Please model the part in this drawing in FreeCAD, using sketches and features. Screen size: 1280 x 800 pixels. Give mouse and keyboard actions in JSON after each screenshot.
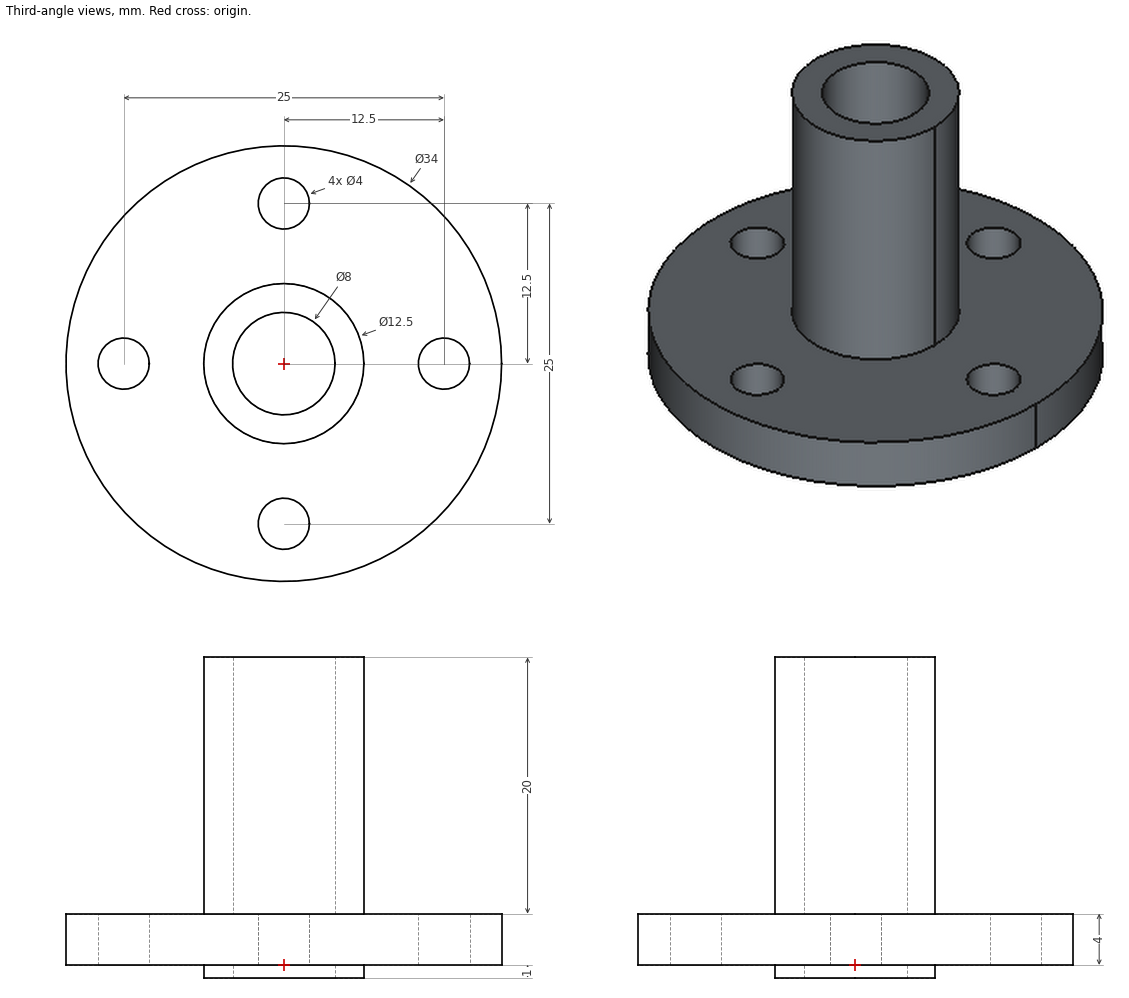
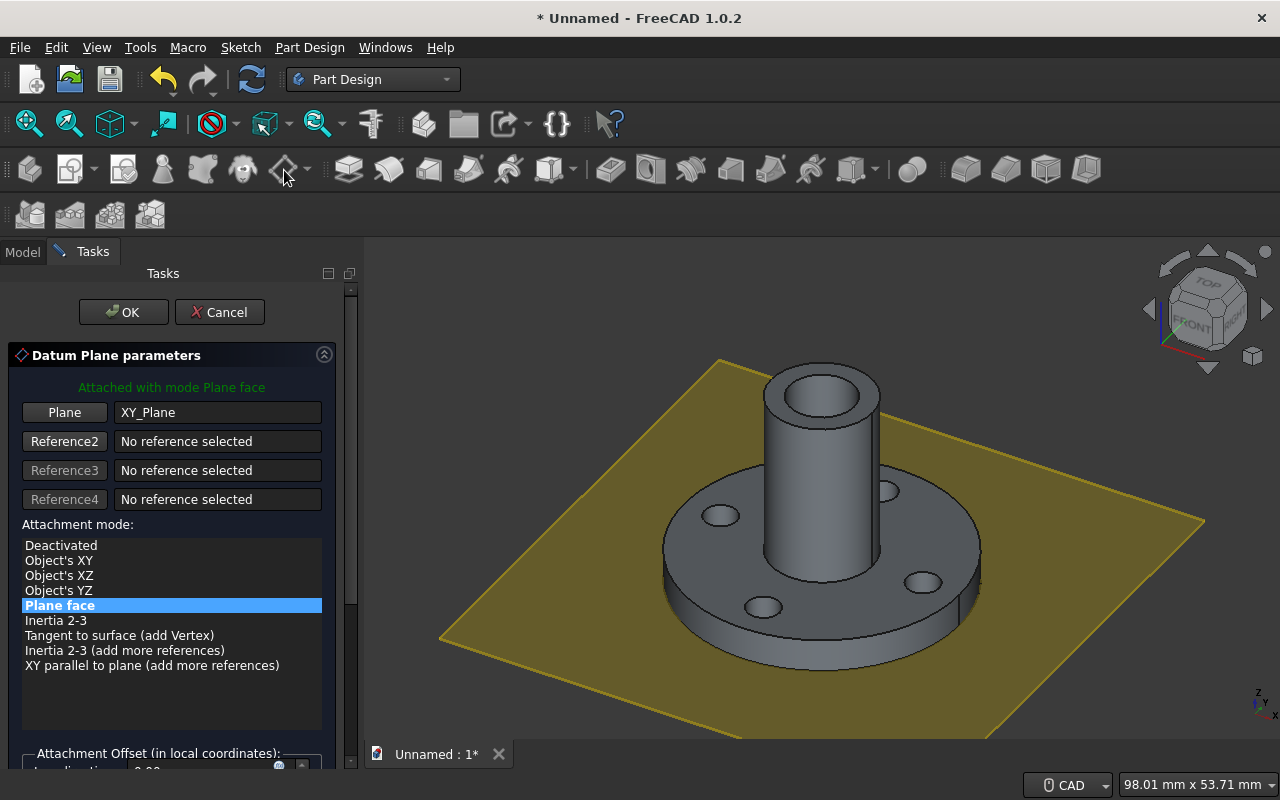
{"action": "scroll", "coordinate": [351, 526], "scroll_direction": "down", "scroll_amount": 3}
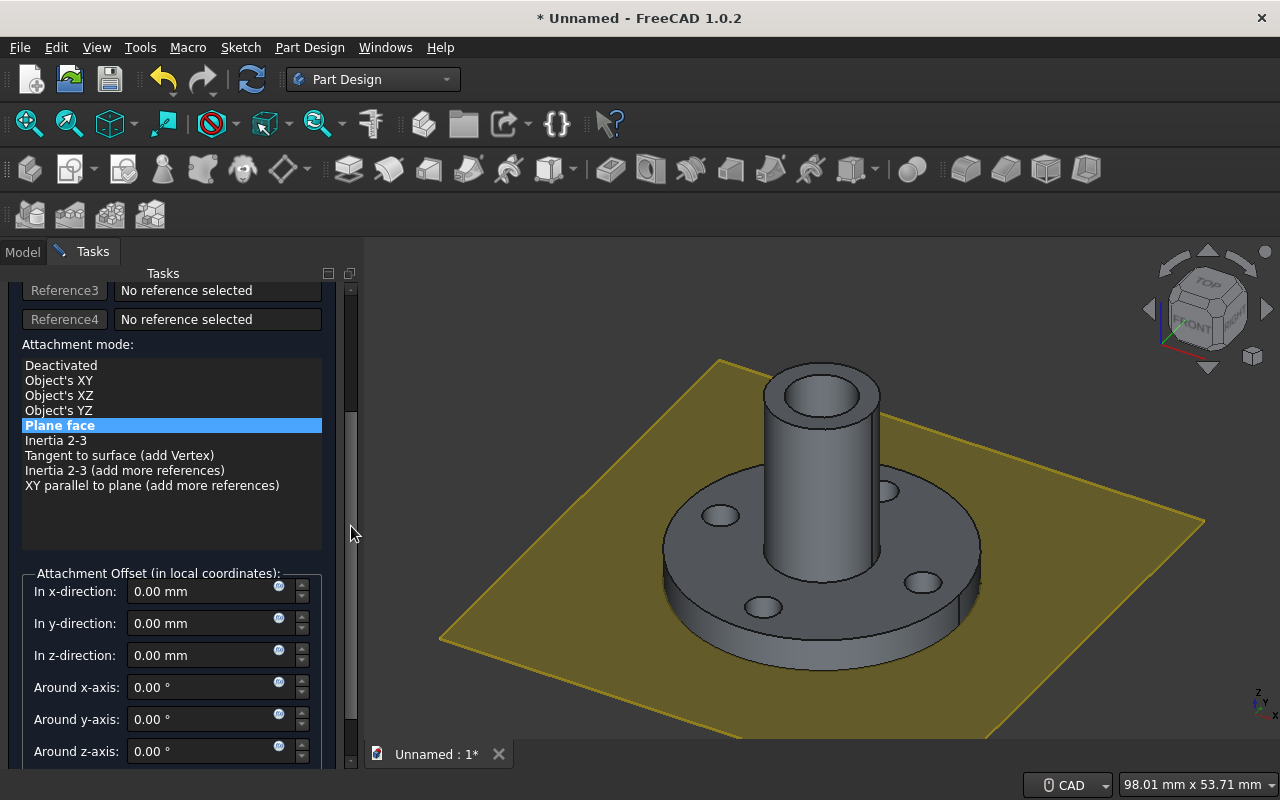
{"action": "triple_click", "coordinate": [210, 655]}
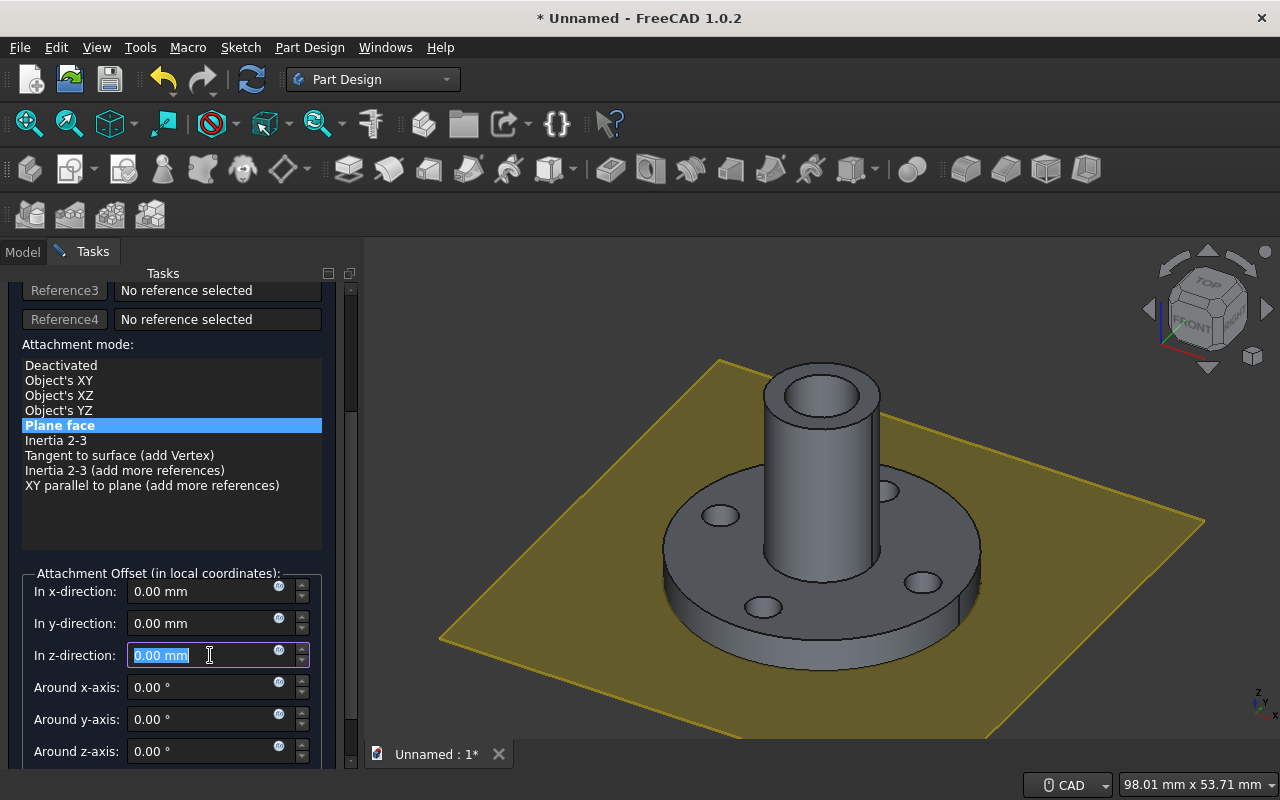
{"action": "type", "text": "-1"}
{"action": "key", "text": "Tab"}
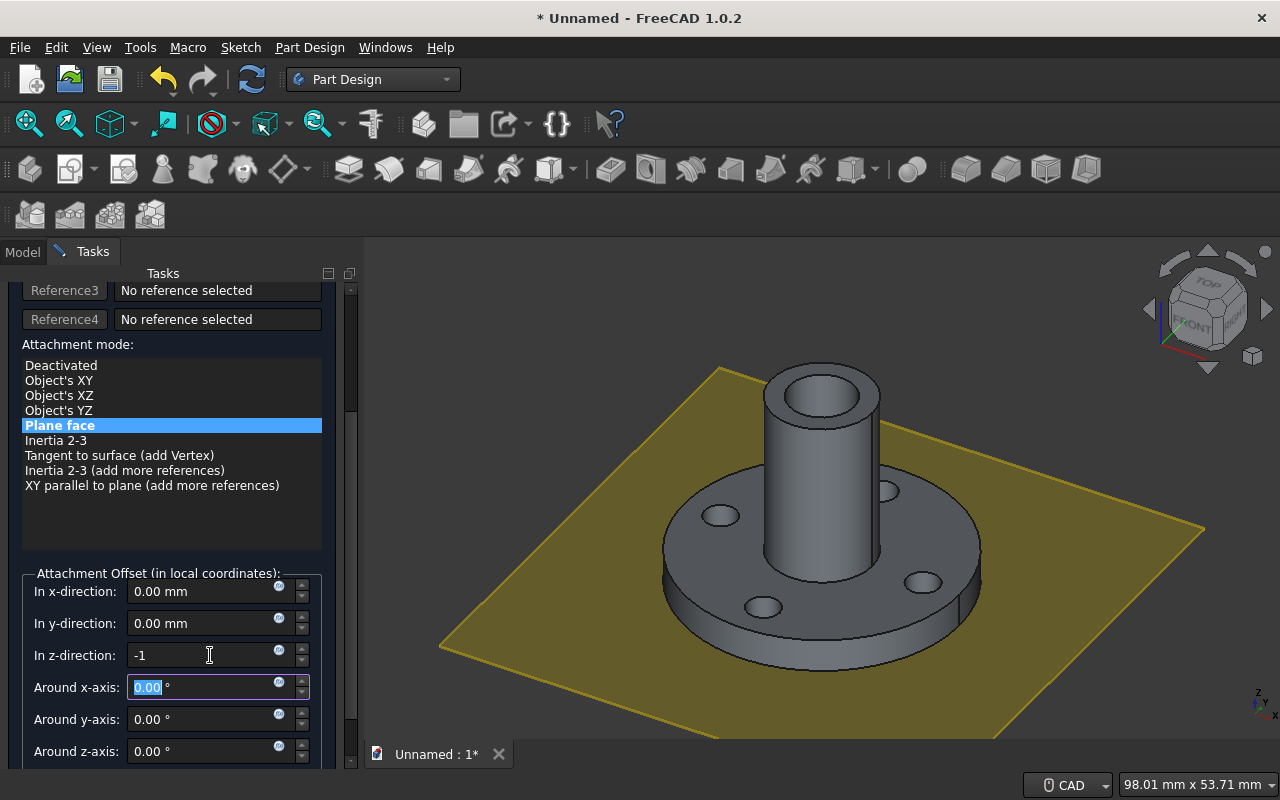
{"action": "scroll", "coordinate": [351, 526], "scroll_direction": "up", "scroll_amount": 4}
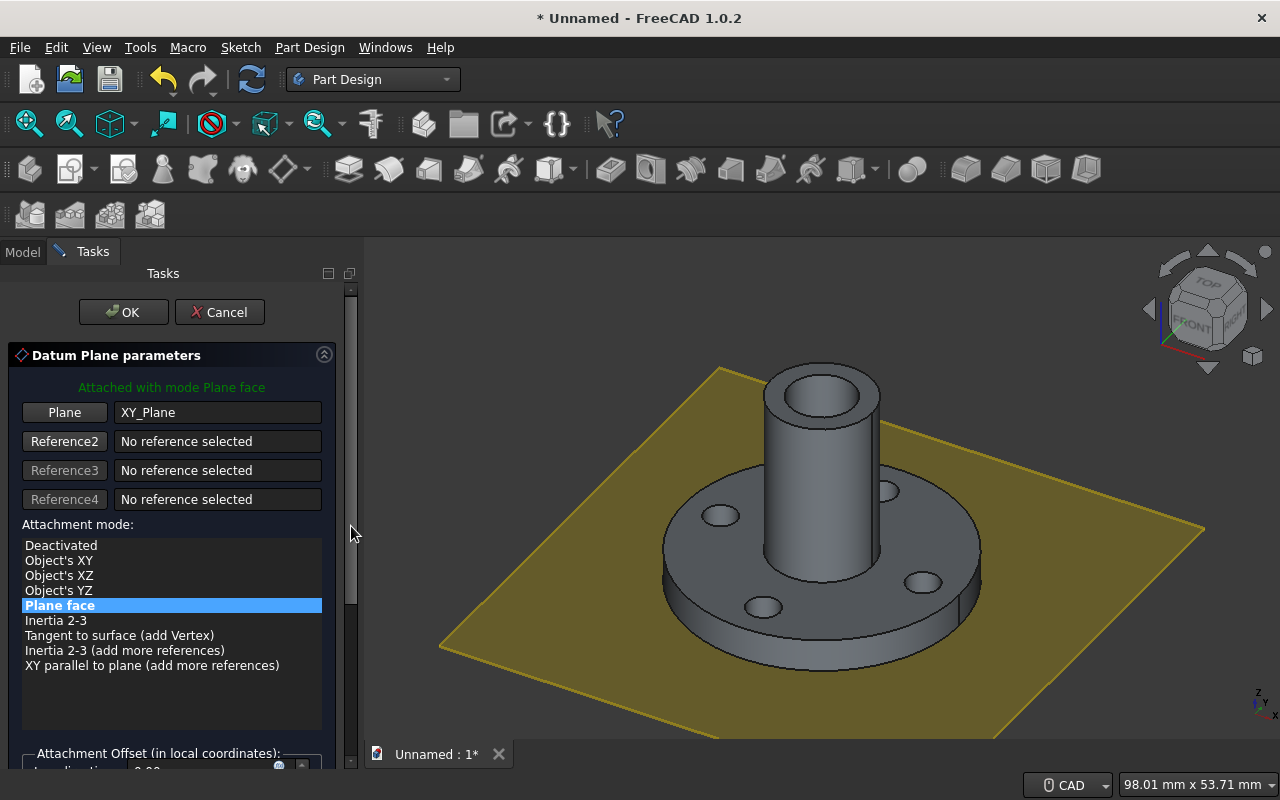
{"action": "left_click", "coordinate": [124, 312]}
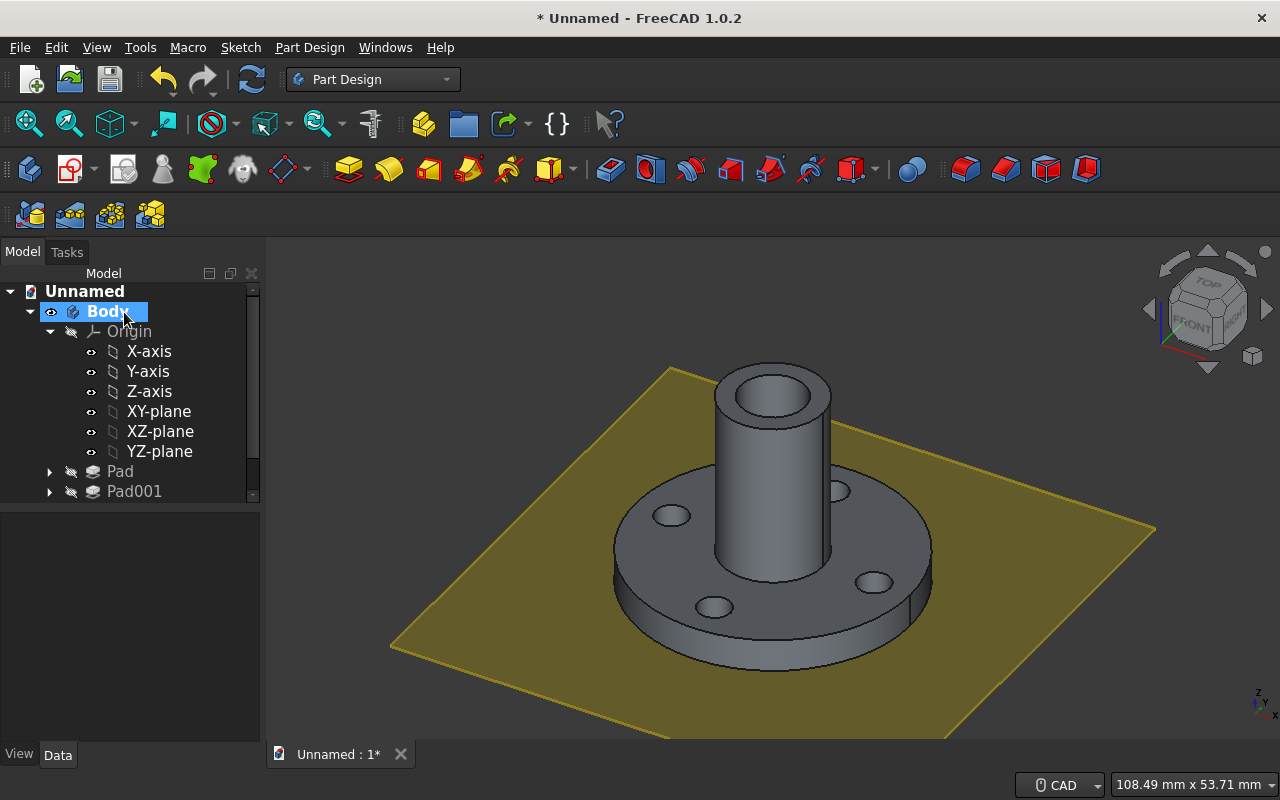
{"action": "scroll", "coordinate": [100, 387], "scroll_direction": "down", "scroll_amount": 3}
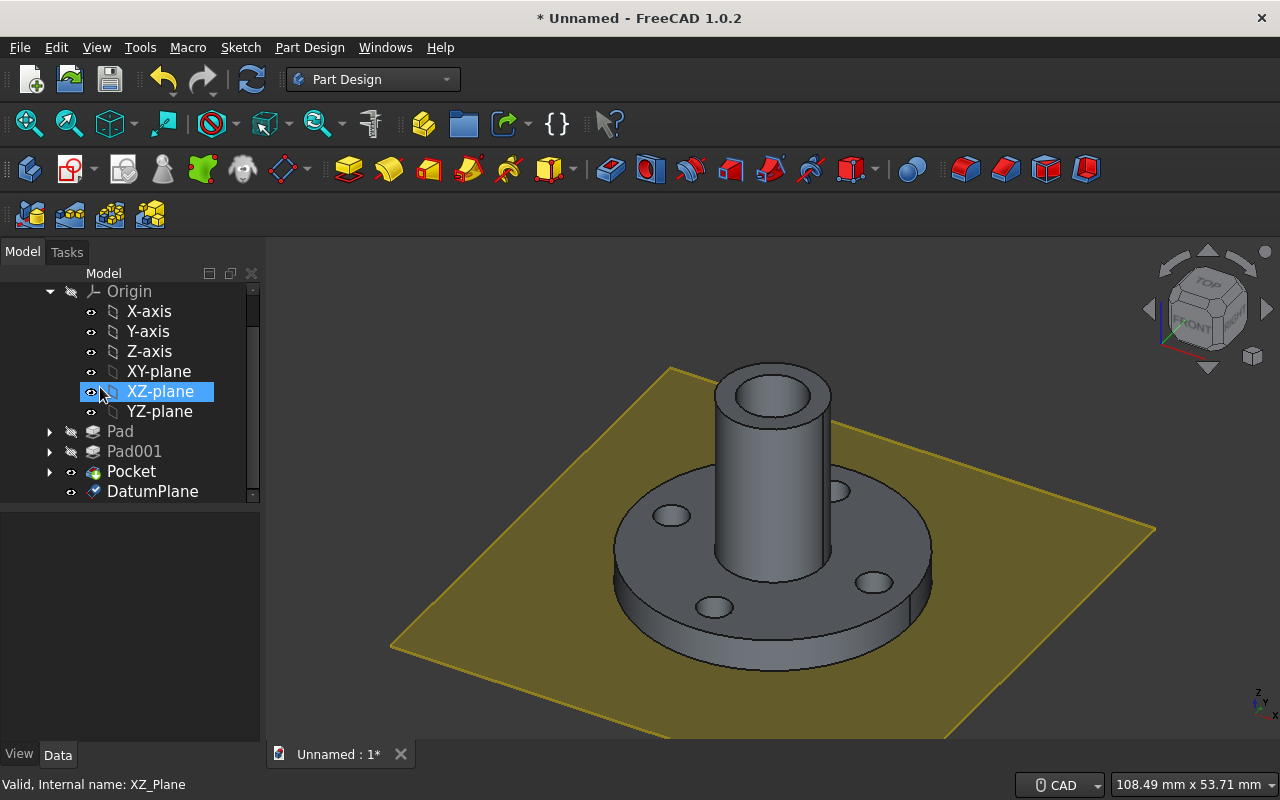
{"action": "left_click", "coordinate": [116, 492]}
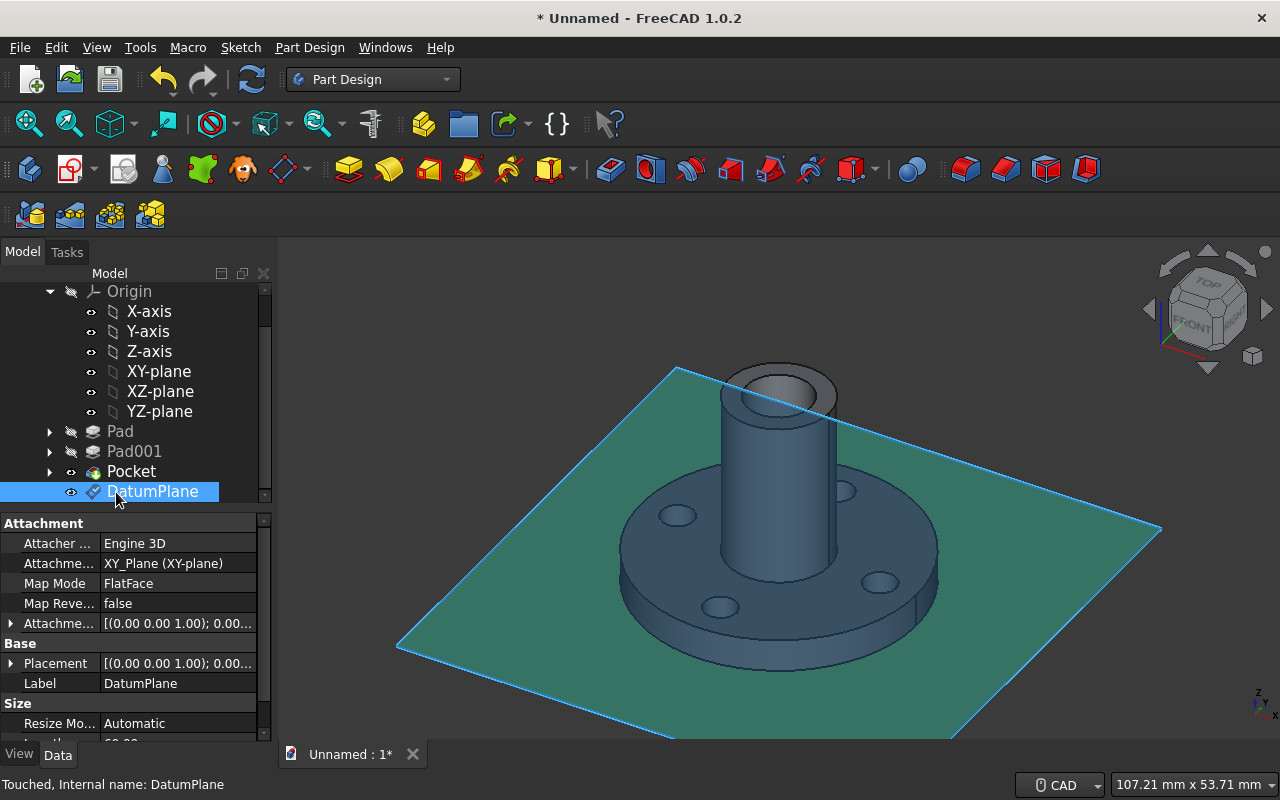
{"action": "left_click", "coordinate": [70, 170]}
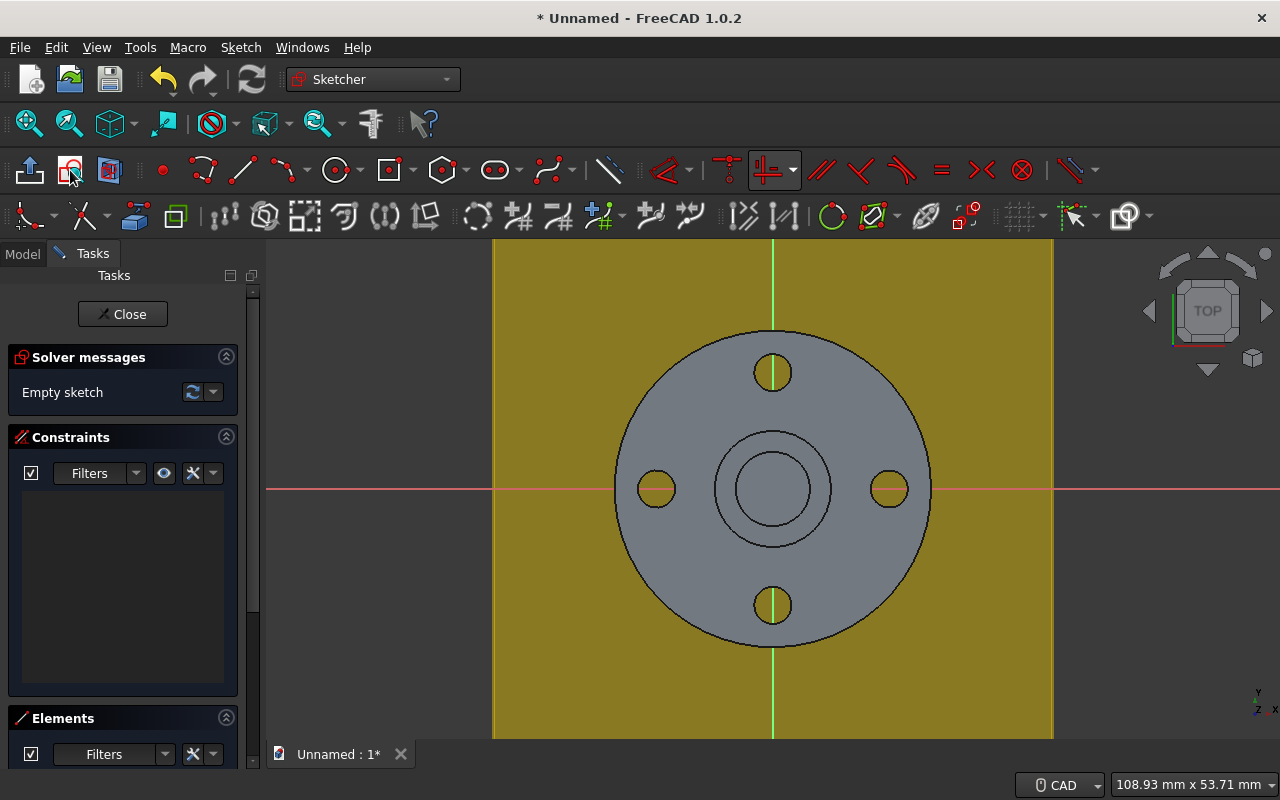
{"action": "left_click", "coordinate": [110, 170]}